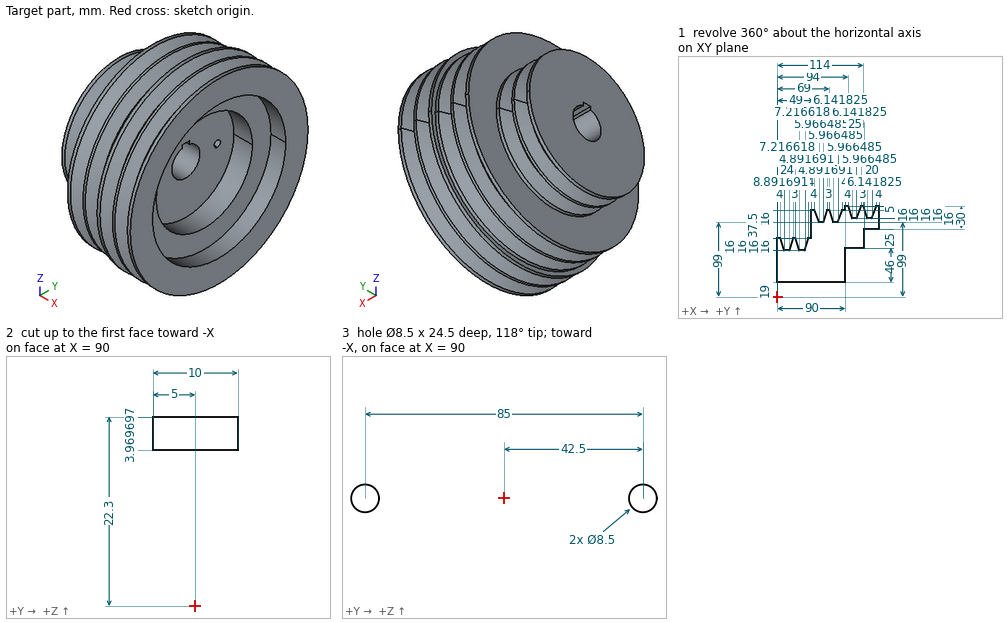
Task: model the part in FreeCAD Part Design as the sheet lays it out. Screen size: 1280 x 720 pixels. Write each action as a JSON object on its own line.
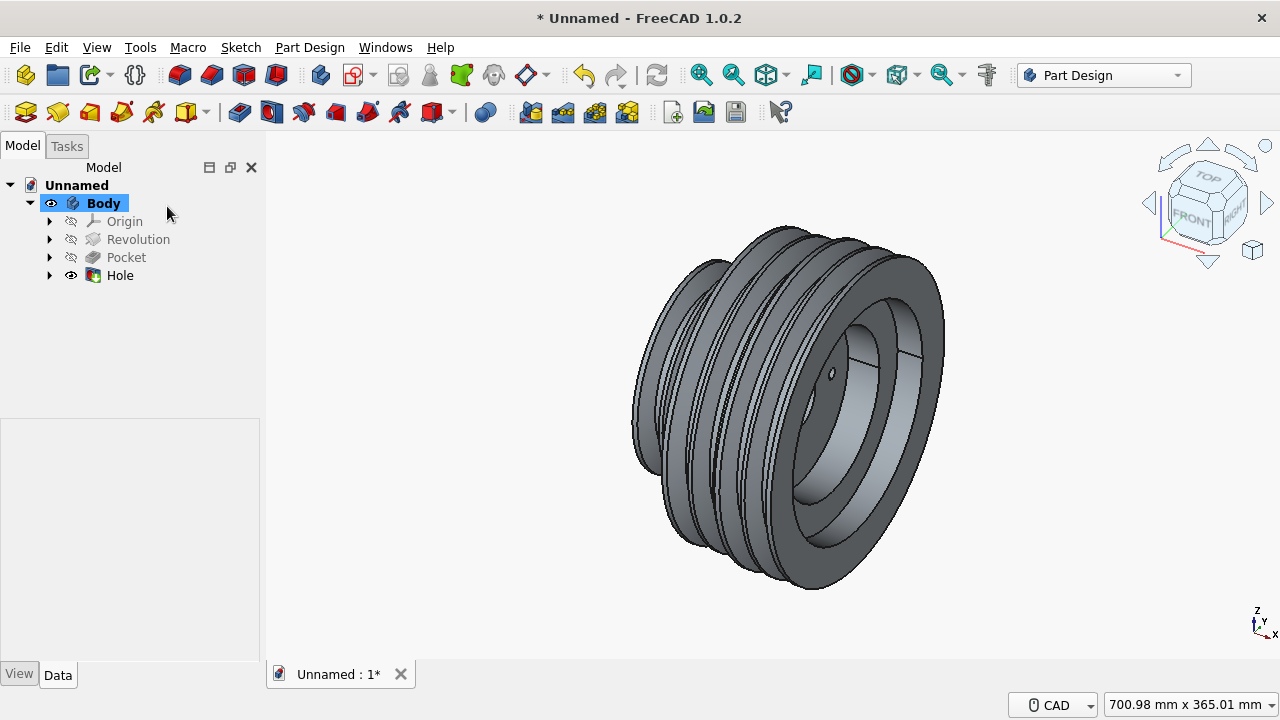
{"action": "key", "text": "0"}